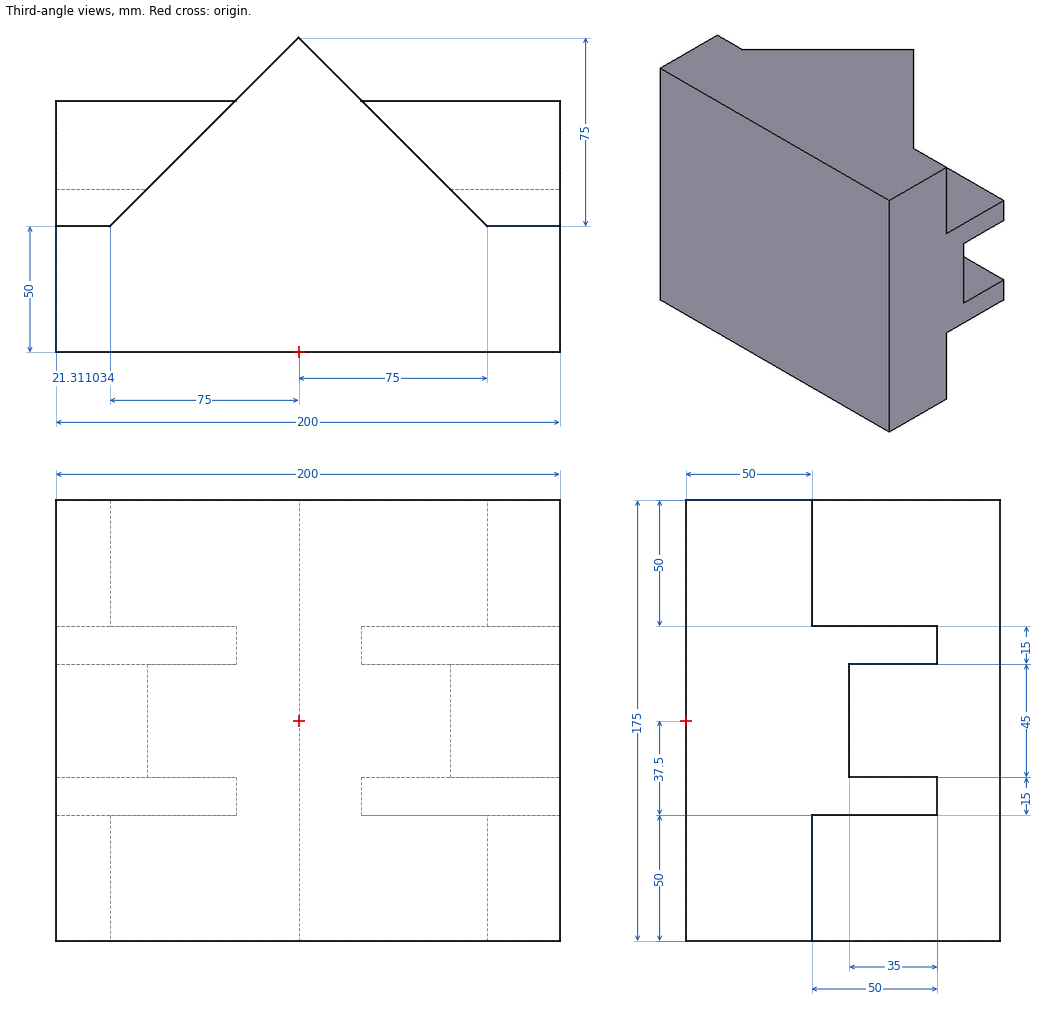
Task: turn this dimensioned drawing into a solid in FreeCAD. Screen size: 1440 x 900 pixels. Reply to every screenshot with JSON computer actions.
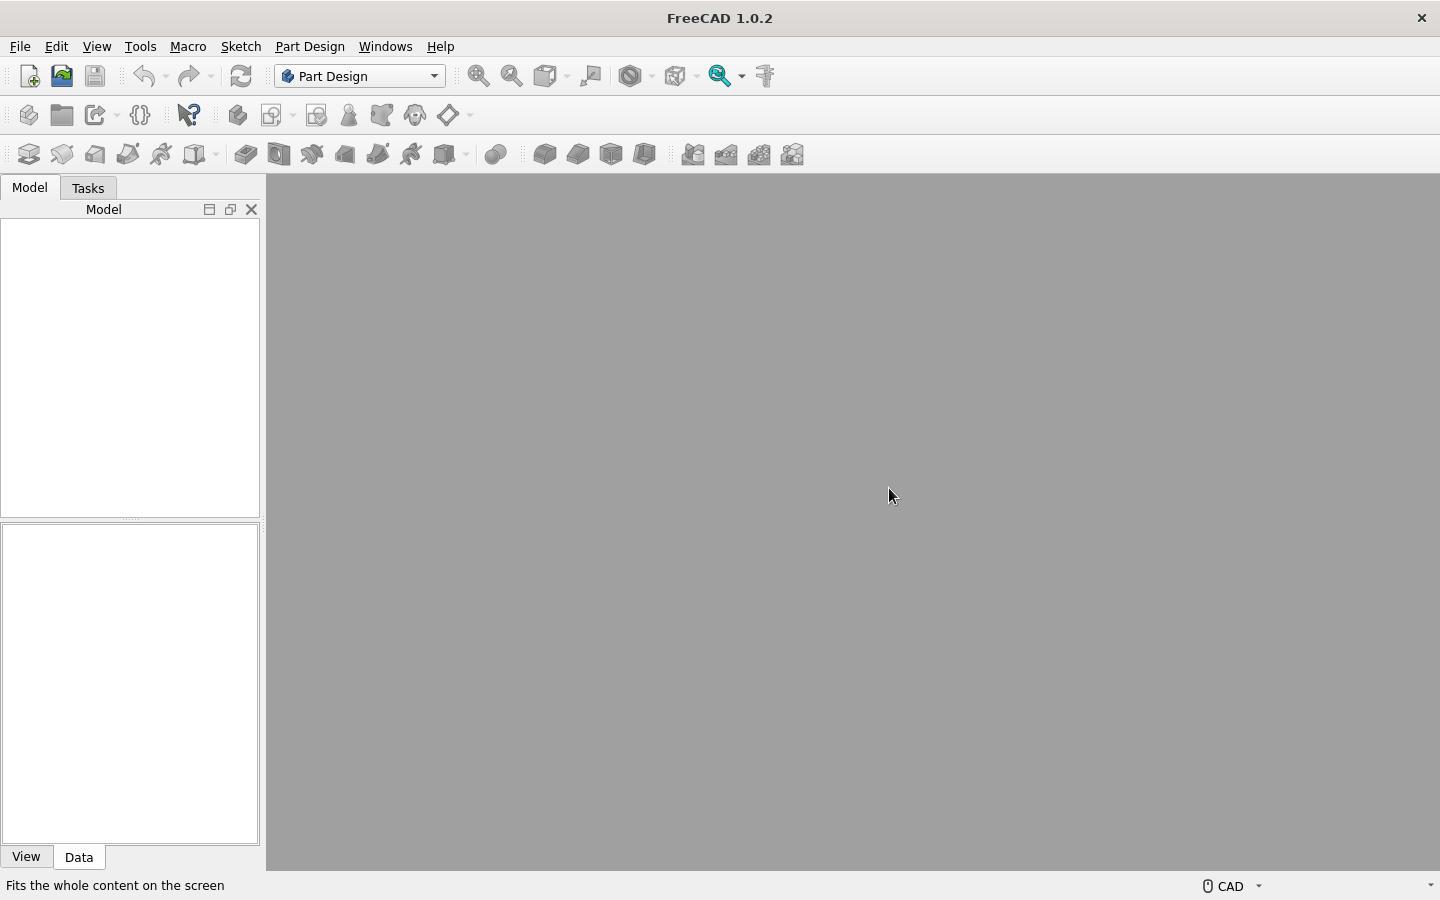
{"action": "left_click", "coordinate": [29, 76]}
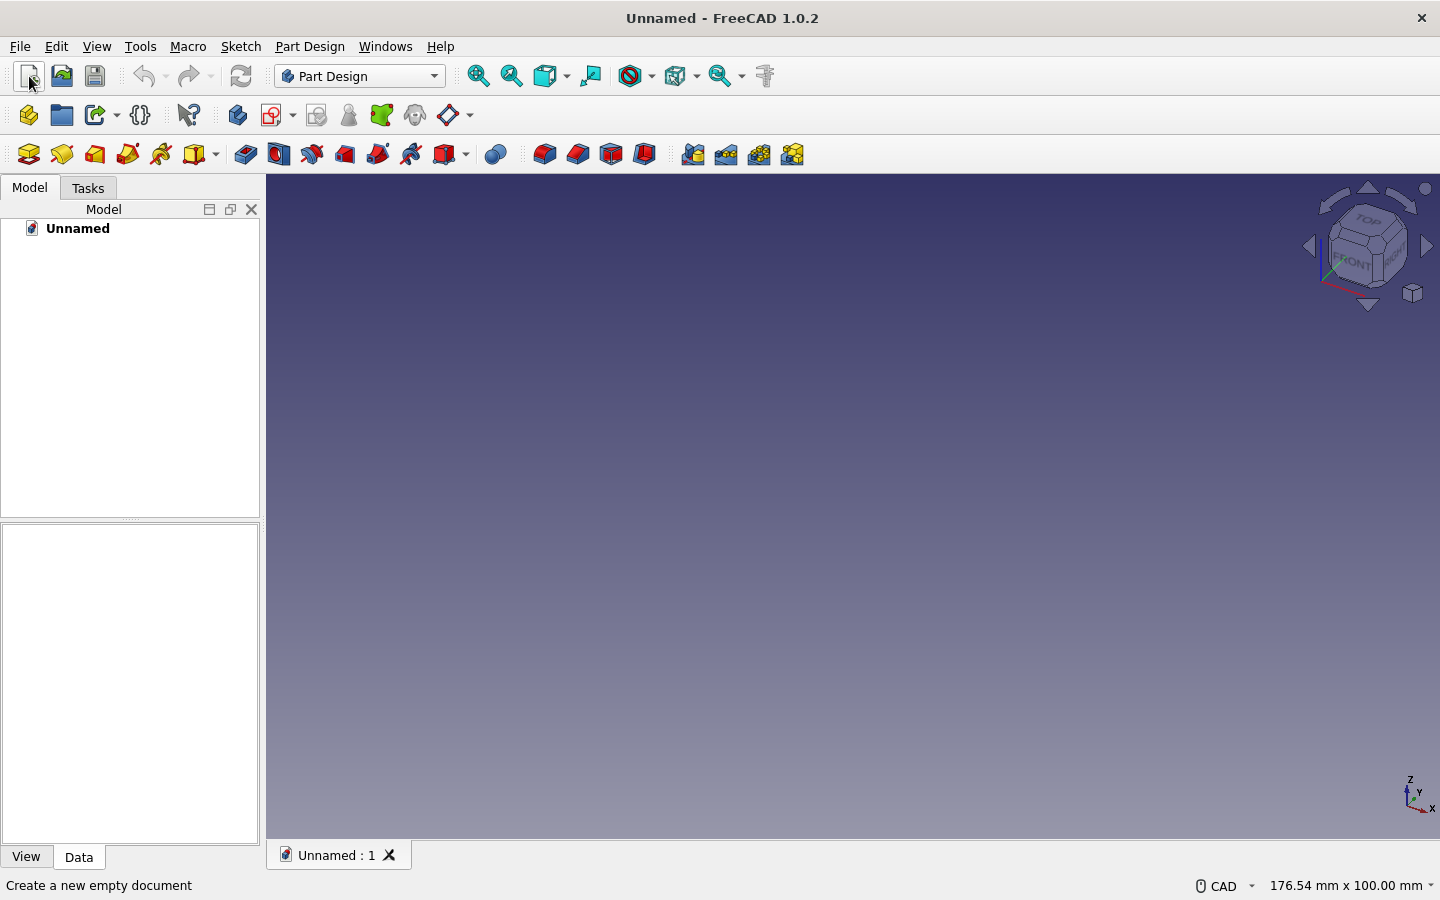
{"action": "left_click", "coordinate": [270, 116]}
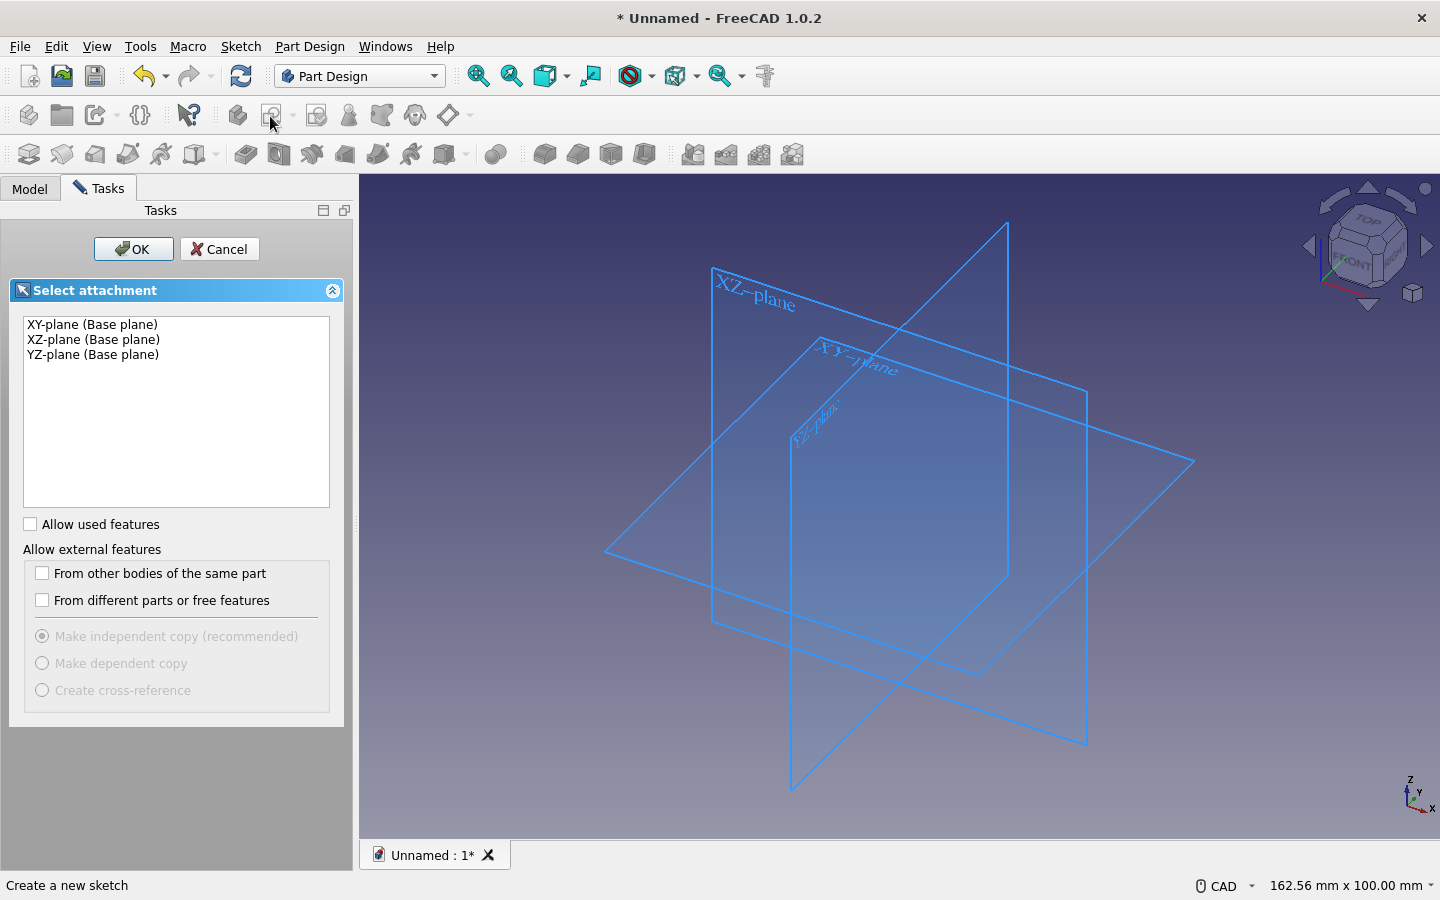
{"action": "left_click", "coordinate": [84, 324]}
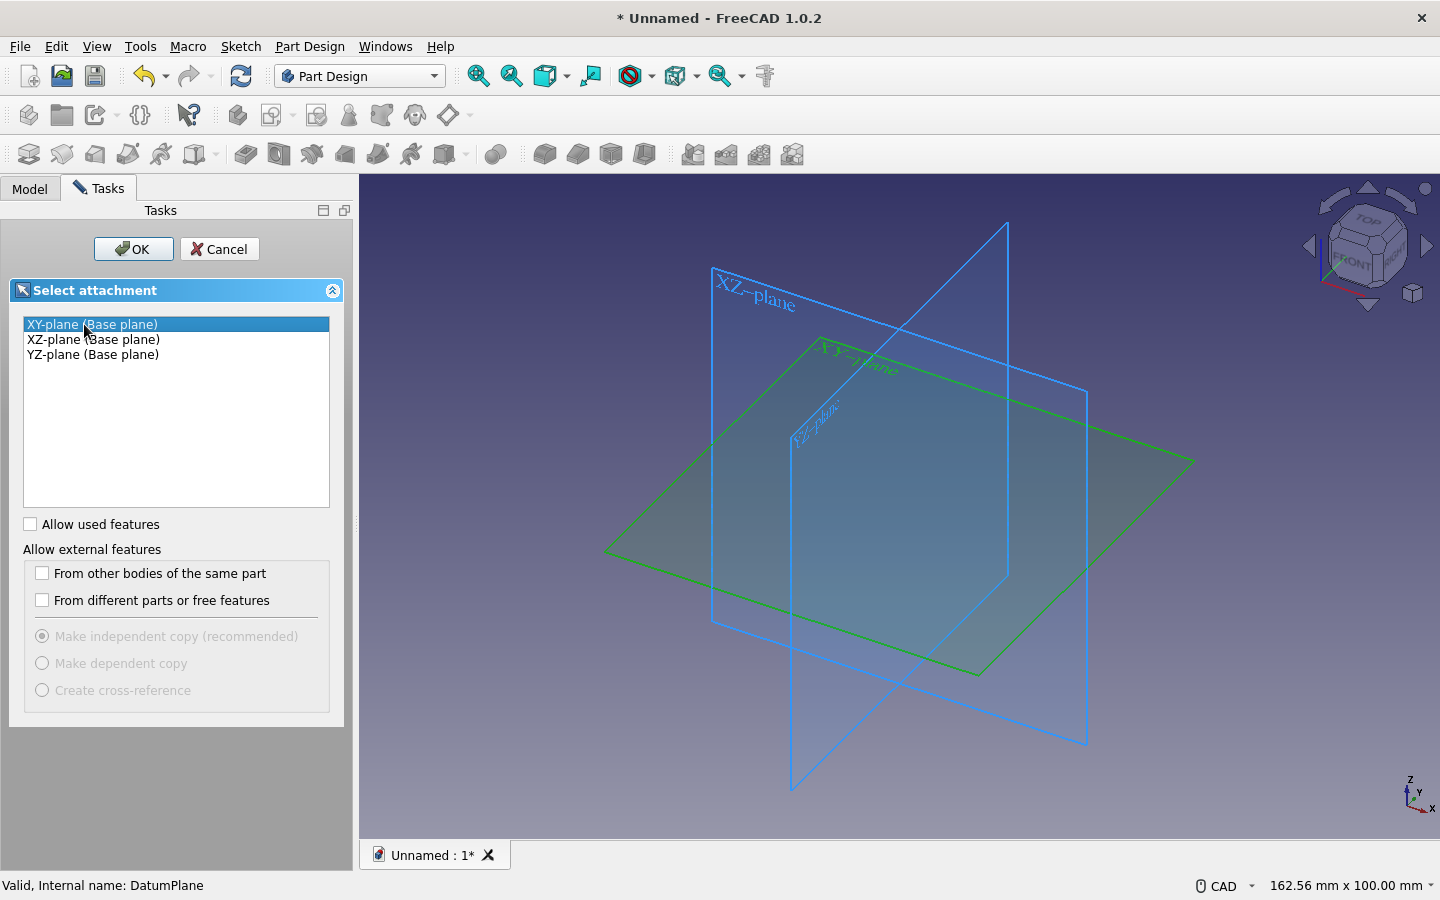
{"action": "left_click", "coordinate": [134, 249]}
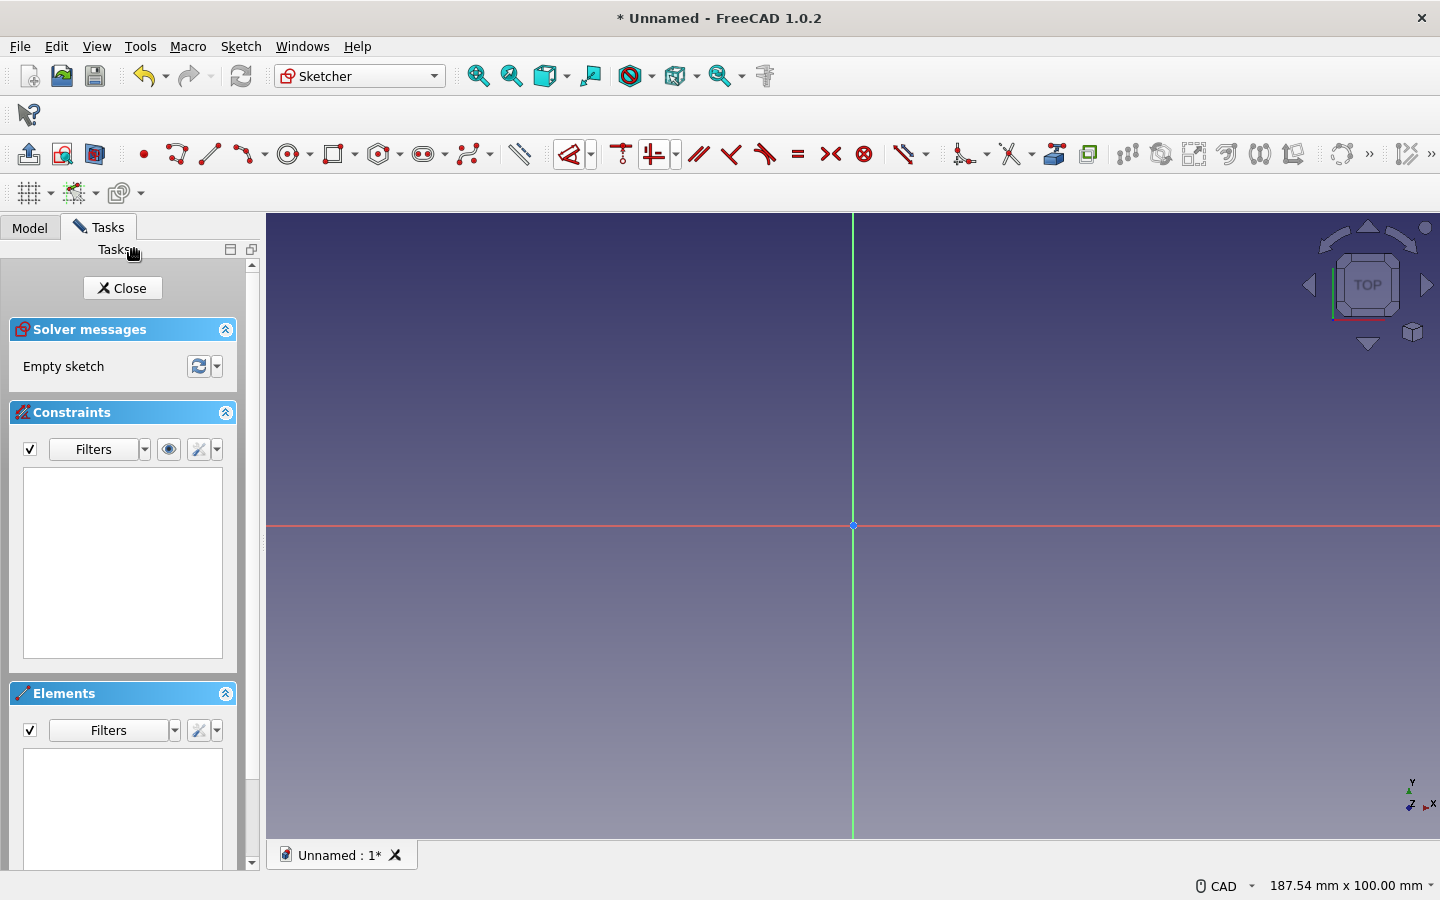
{"action": "scroll", "coordinate": [710, 811], "scroll_direction": "down", "scroll_amount": 4}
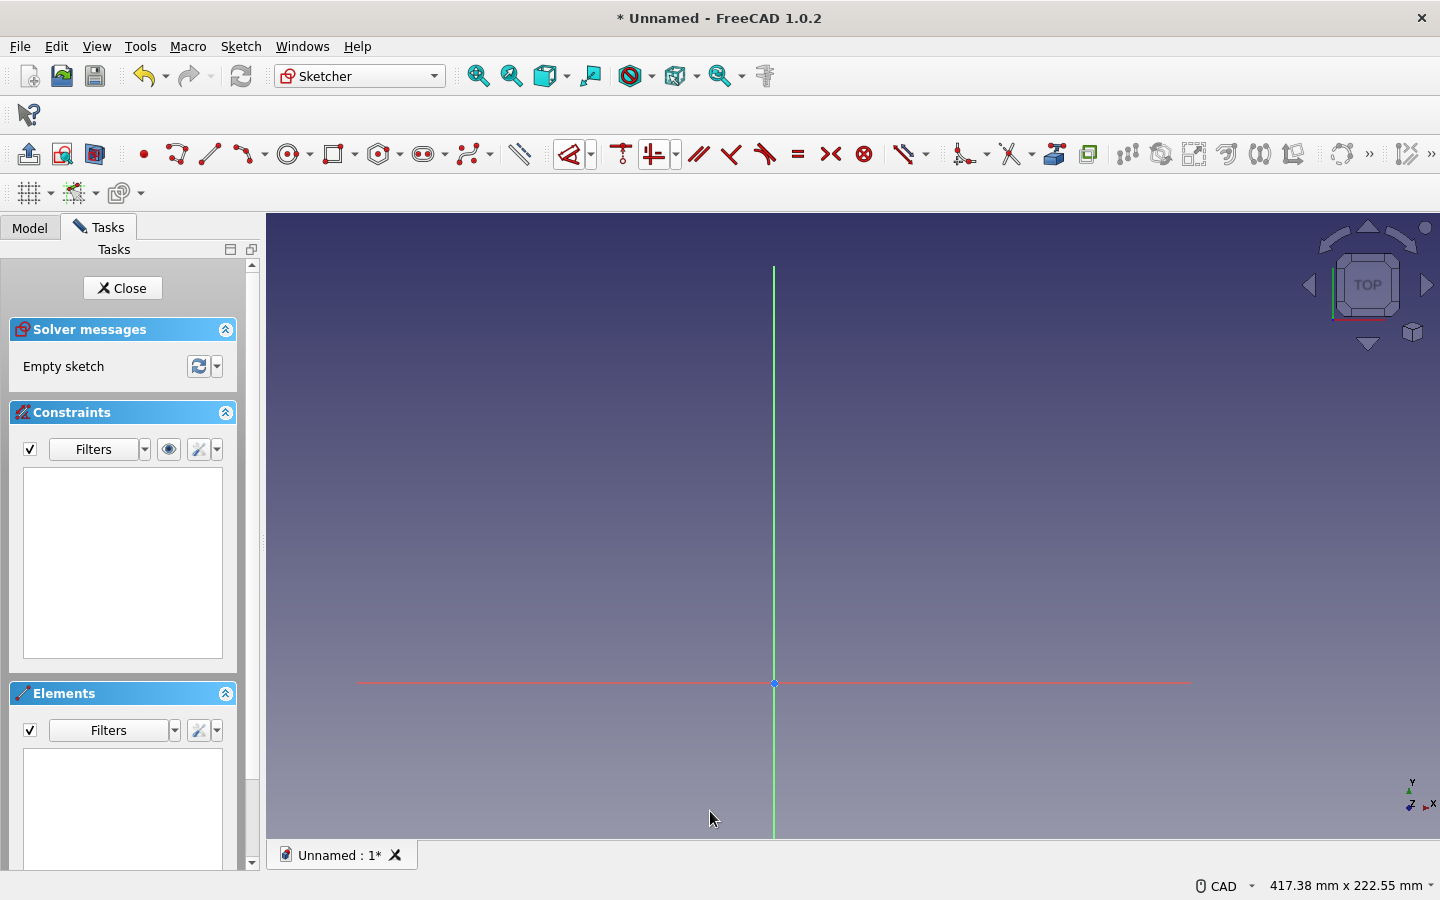
{"action": "left_click", "coordinate": [177, 154]}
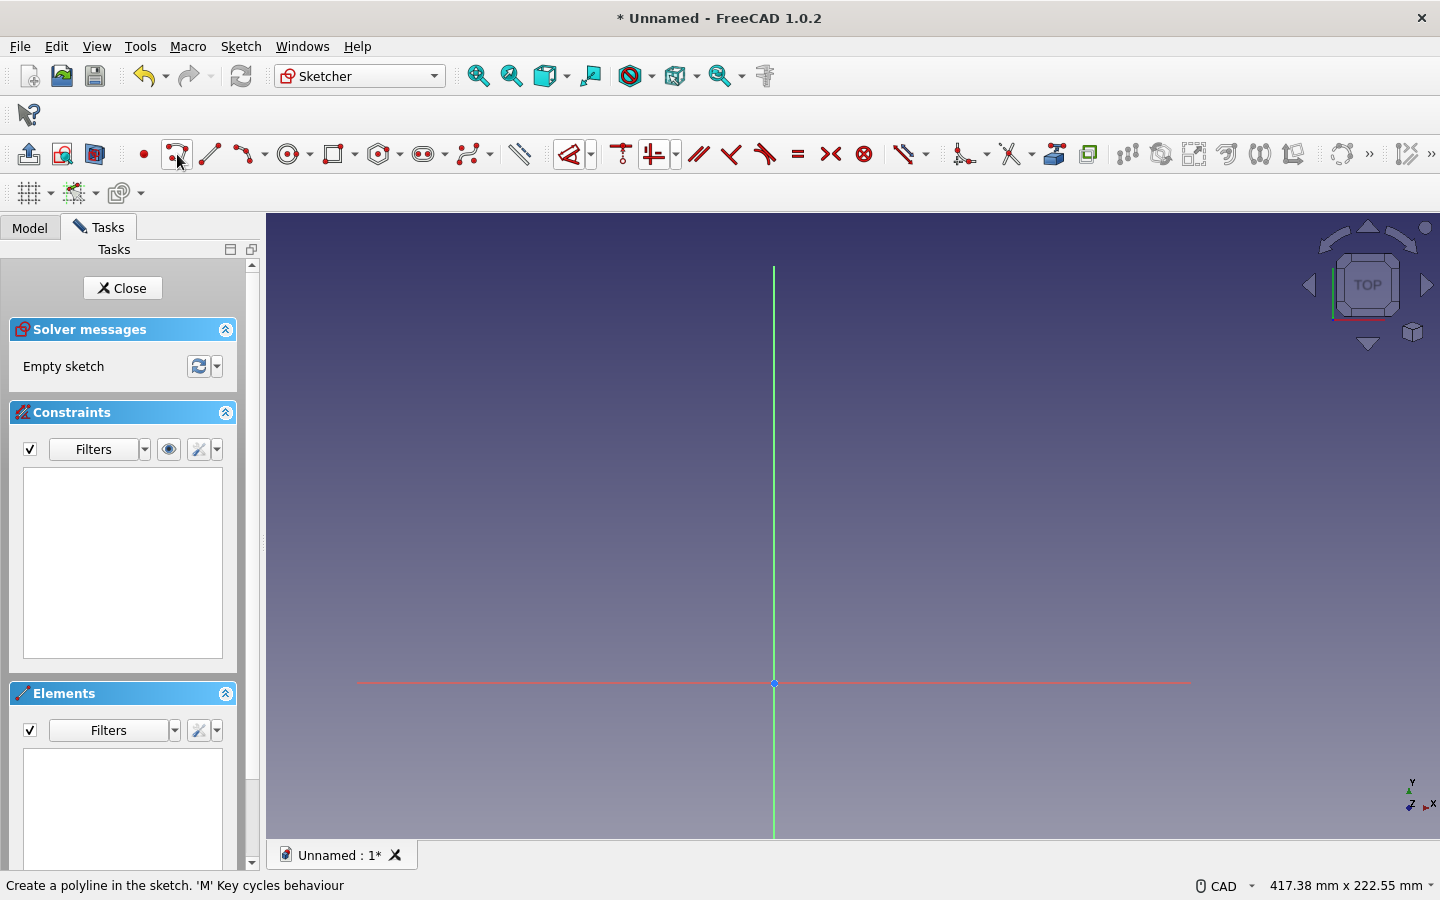
{"action": "left_click", "coordinate": [985, 543]}
{"action": "left_click", "coordinate": [774, 332]}
{"action": "left_click", "coordinate": [564, 543]}
{"action": "left_click", "coordinate": [504, 543]}
{"action": "left_click", "coordinate": [504, 683]}
{"action": "left_click", "coordinate": [1066, 674]}
{"action": "left_click", "coordinate": [1066, 543]}
{"action": "left_click", "coordinate": [985, 544]}
{"action": "key", "text": "Escape"}
{"action": "key", "text": "Escape"}